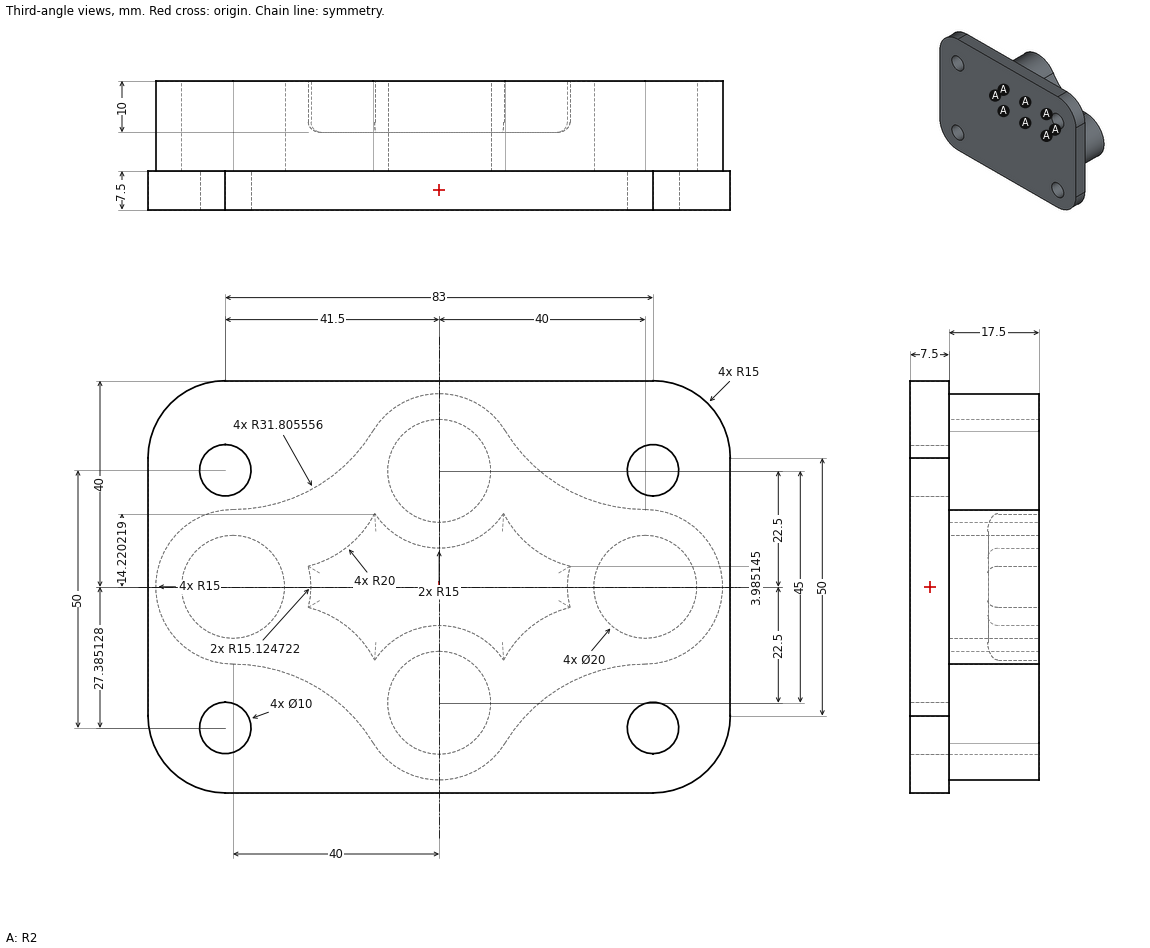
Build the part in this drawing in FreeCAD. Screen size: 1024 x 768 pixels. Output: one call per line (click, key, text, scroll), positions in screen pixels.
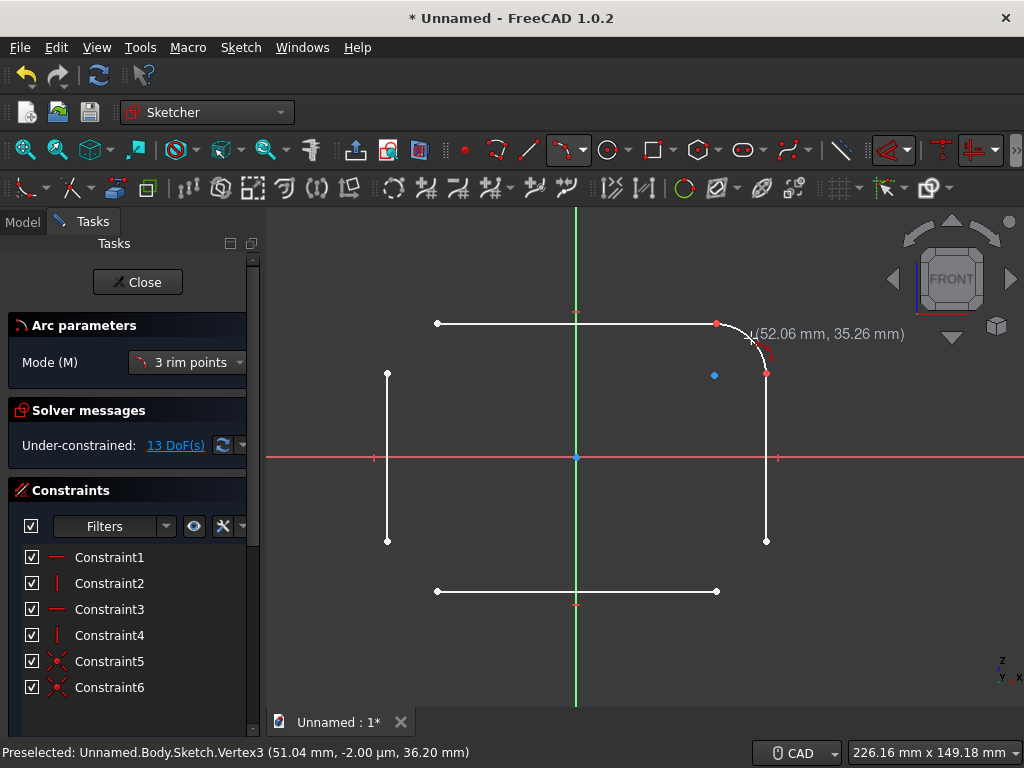
click(766, 542)
click(716, 592)
click(751, 577)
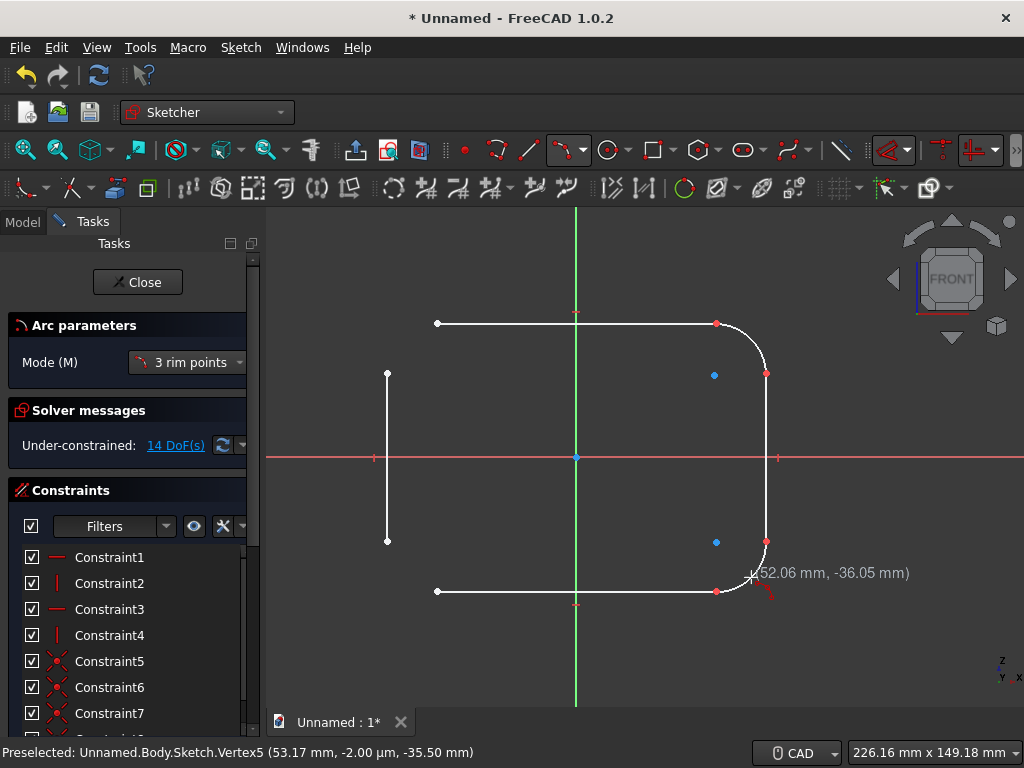
click(437, 592)
click(387, 542)
click(402, 577)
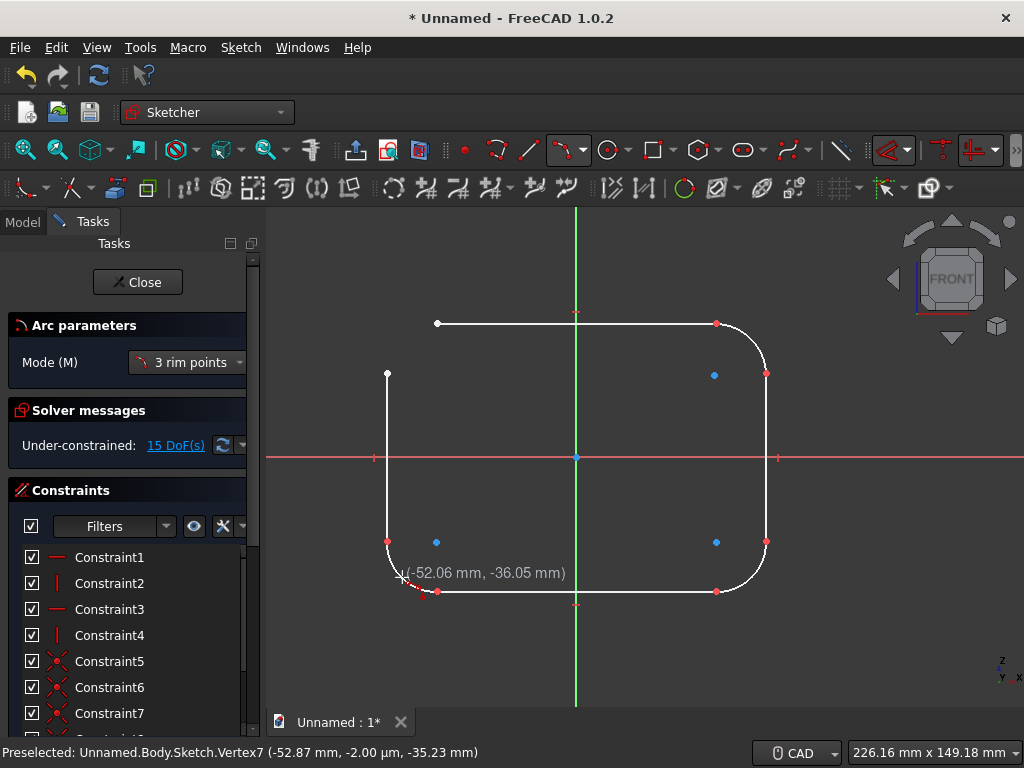
click(387, 374)
click(437, 324)
click(402, 338)
key(Escape)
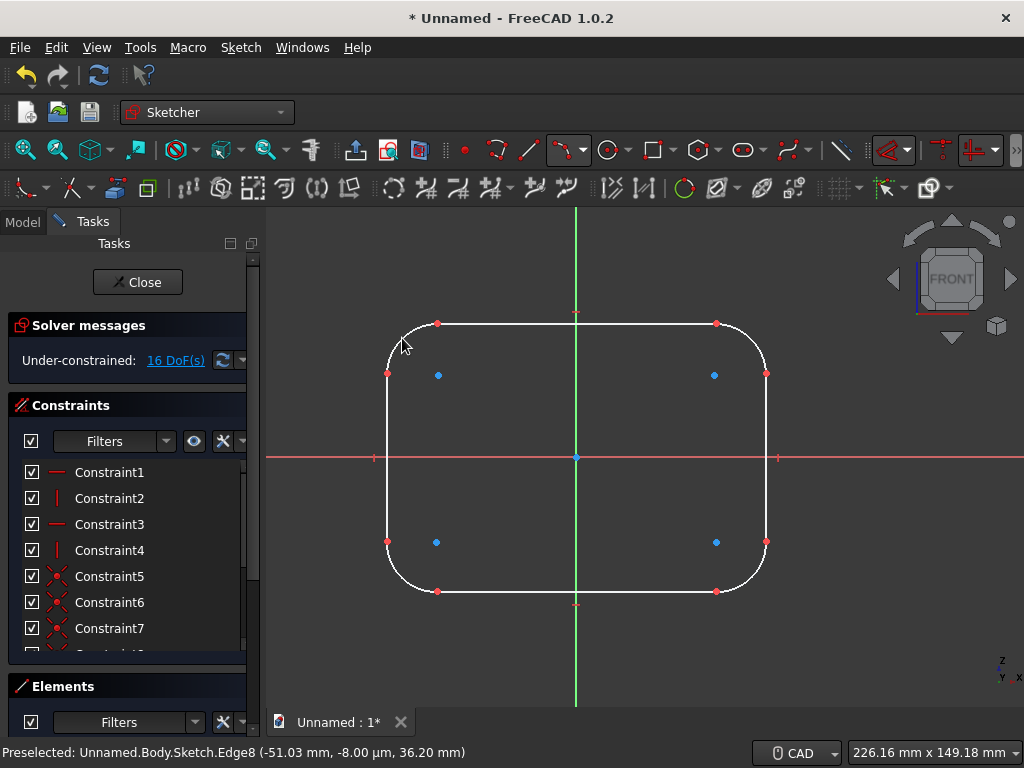
click(521, 324)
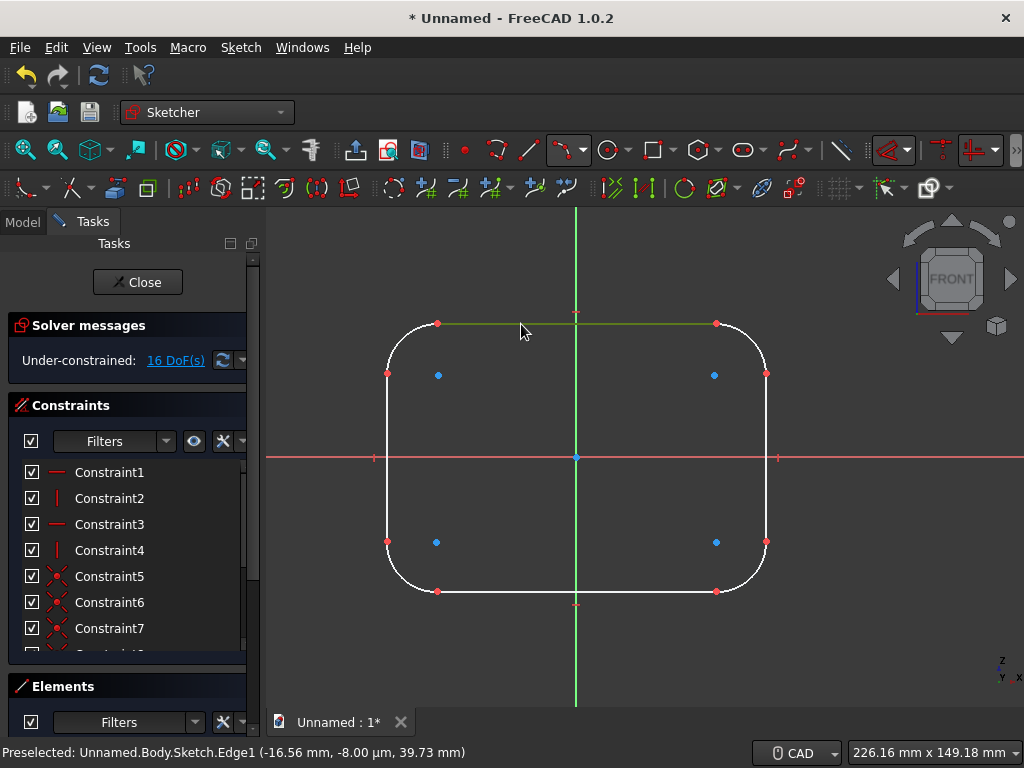
click(760, 352)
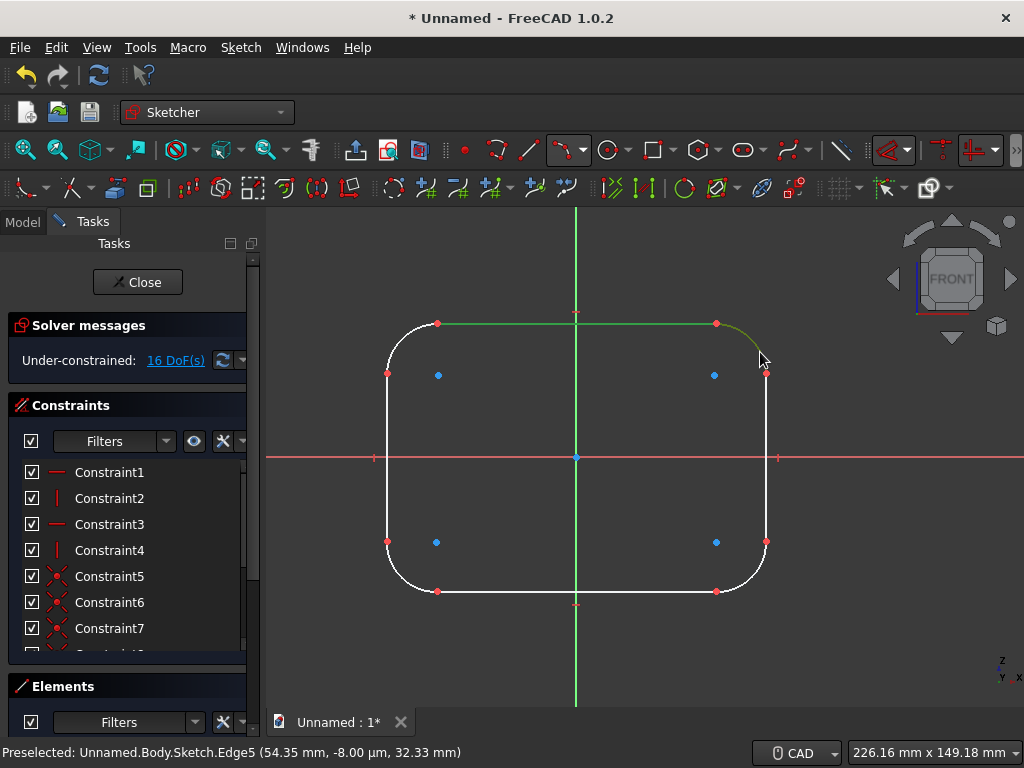
key(t)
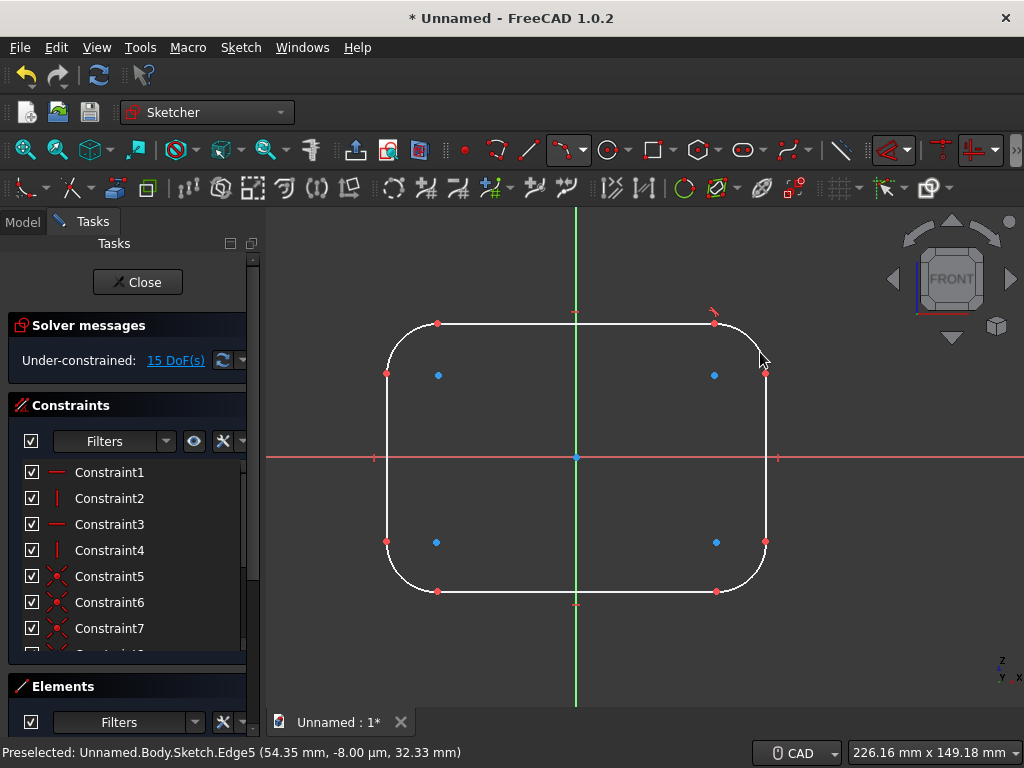
click(520, 324)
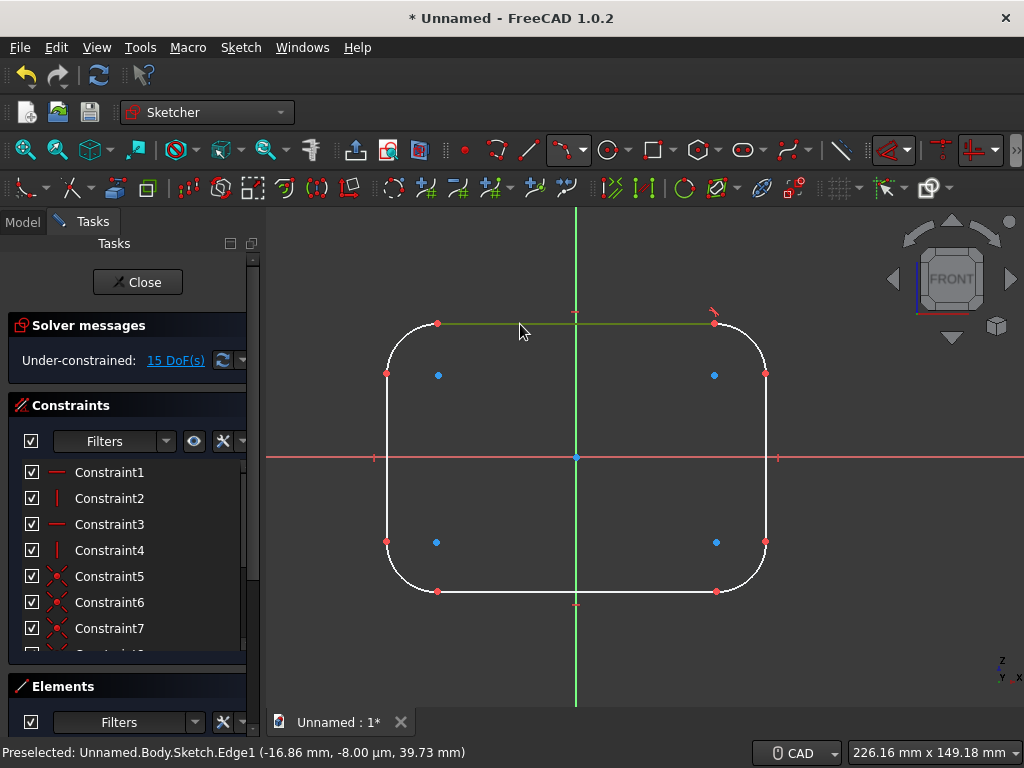
click(415, 330)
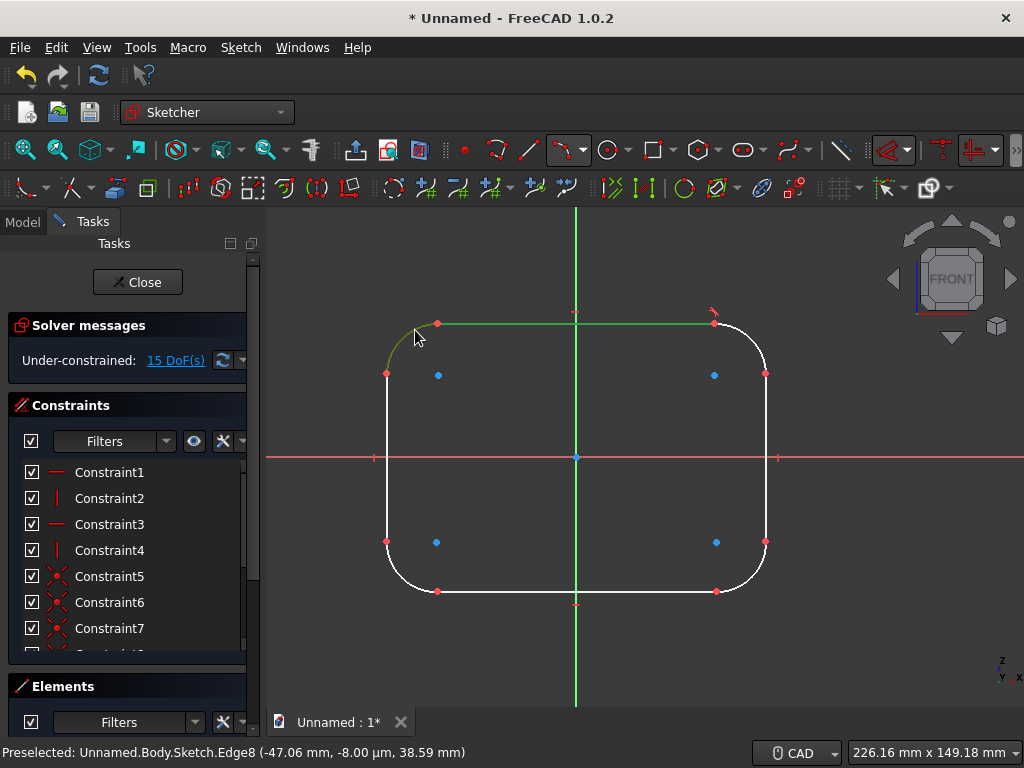
key(t)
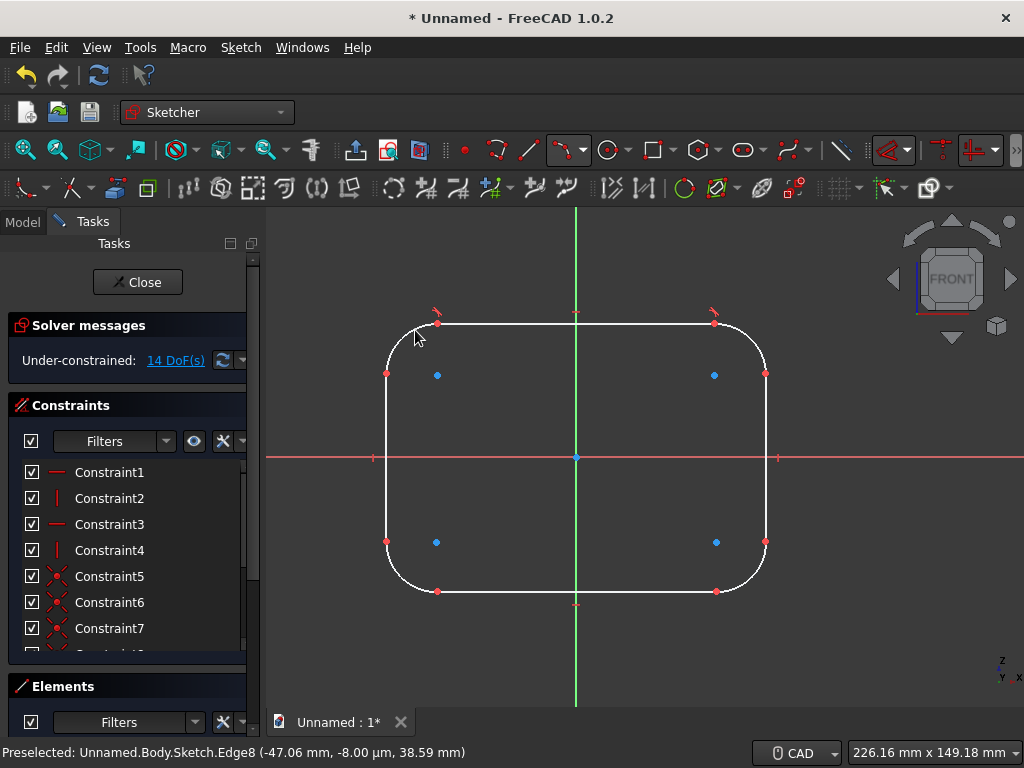
click(766, 424)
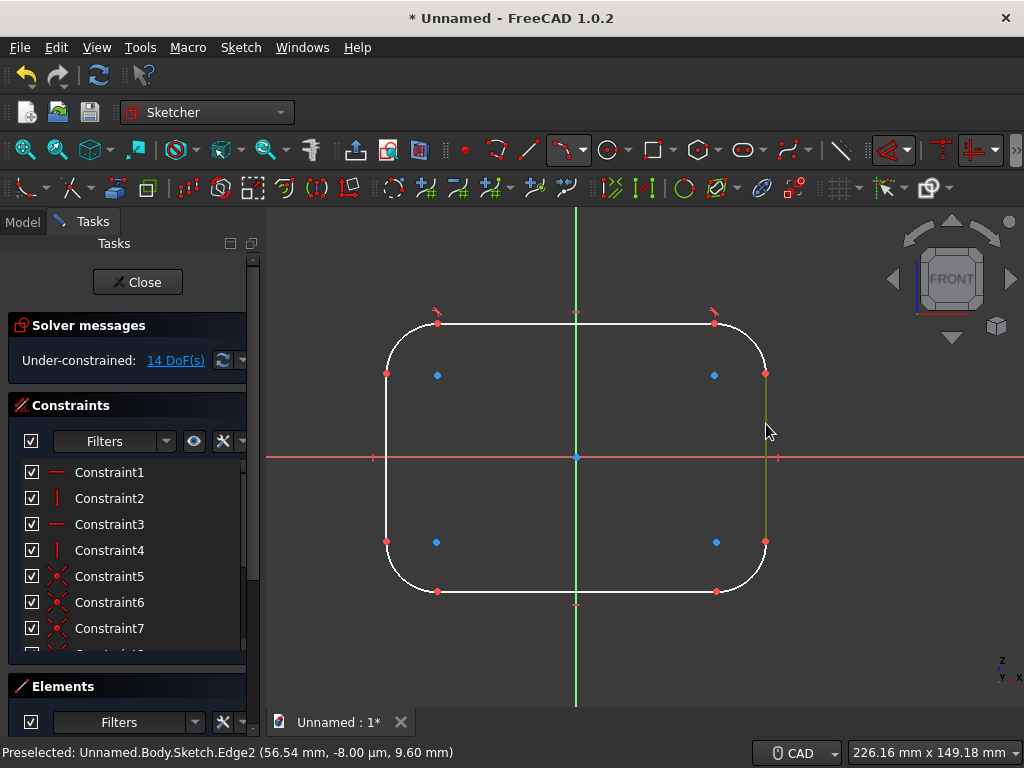
click(760, 351)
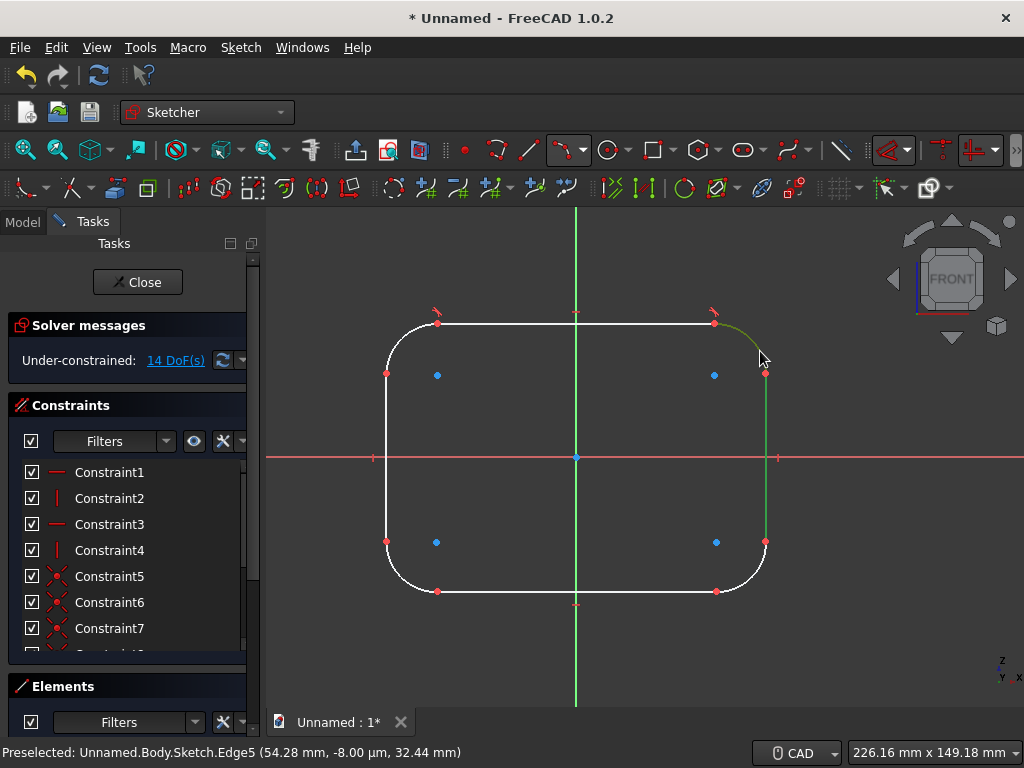
key(t)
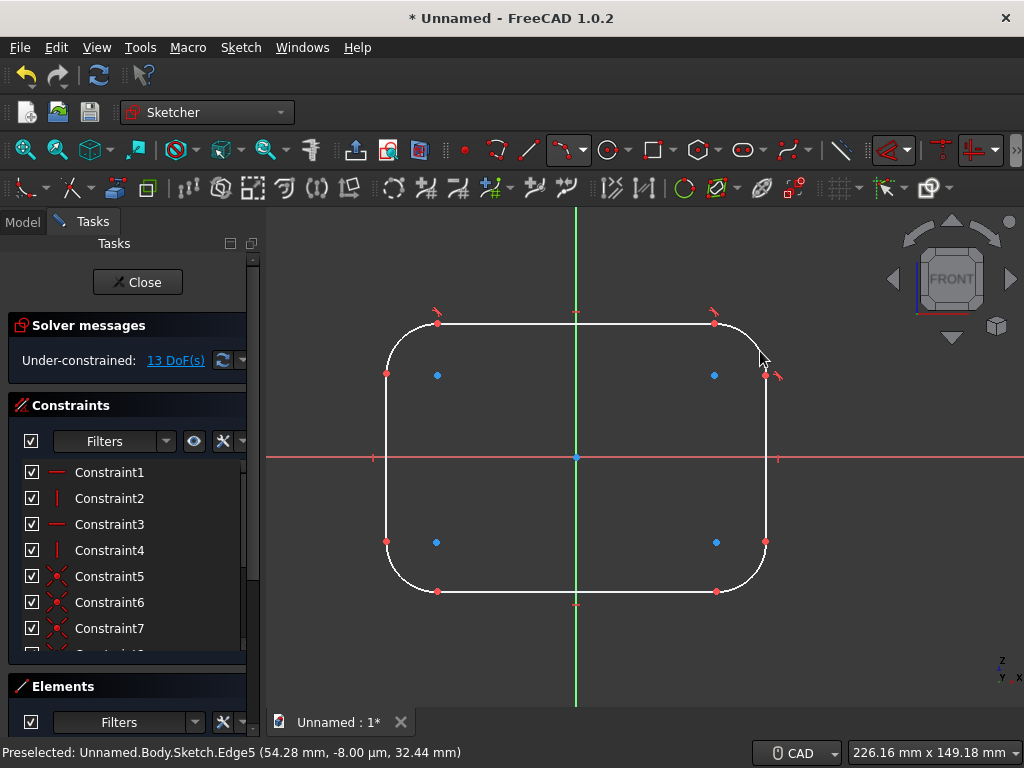
click(766, 425)